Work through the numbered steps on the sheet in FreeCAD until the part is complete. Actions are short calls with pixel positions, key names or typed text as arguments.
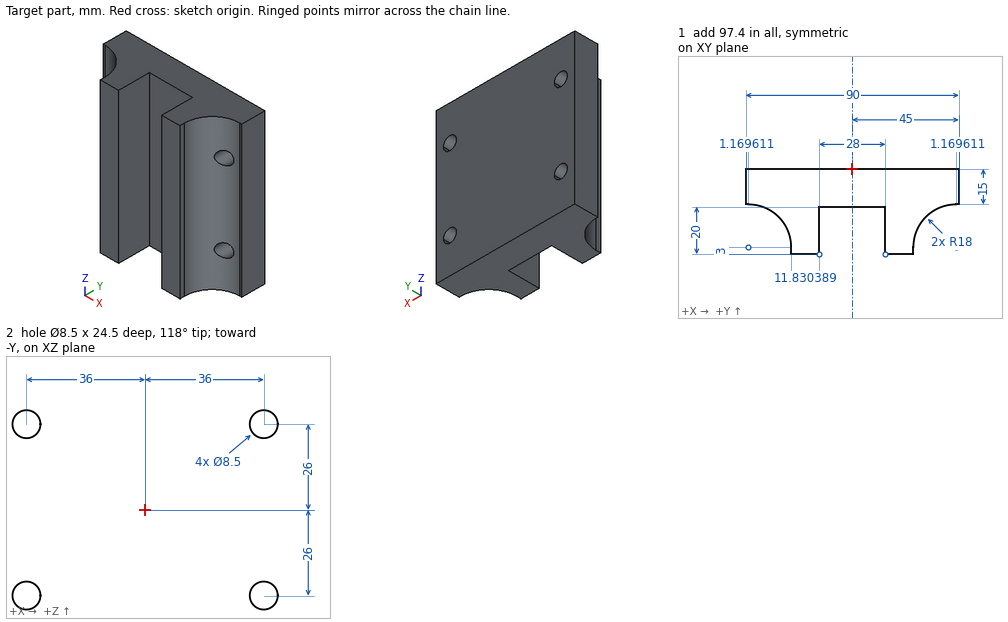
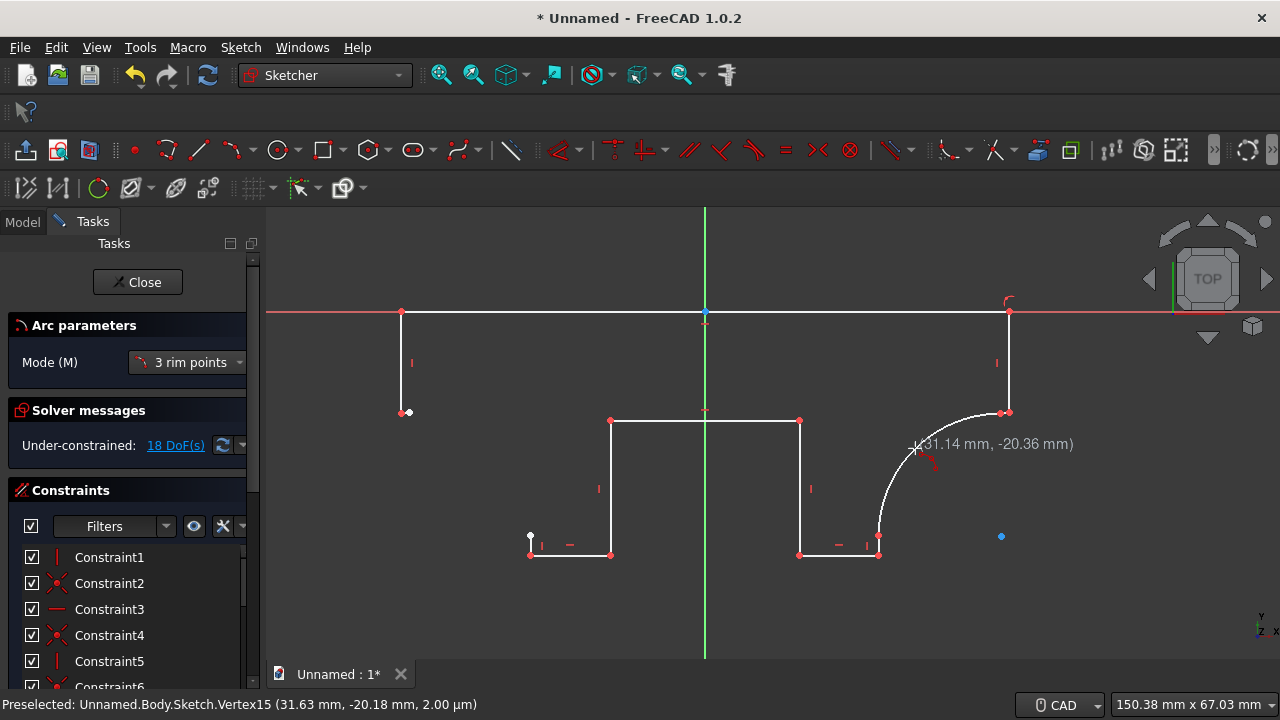
scroll(409, 413, up, 7)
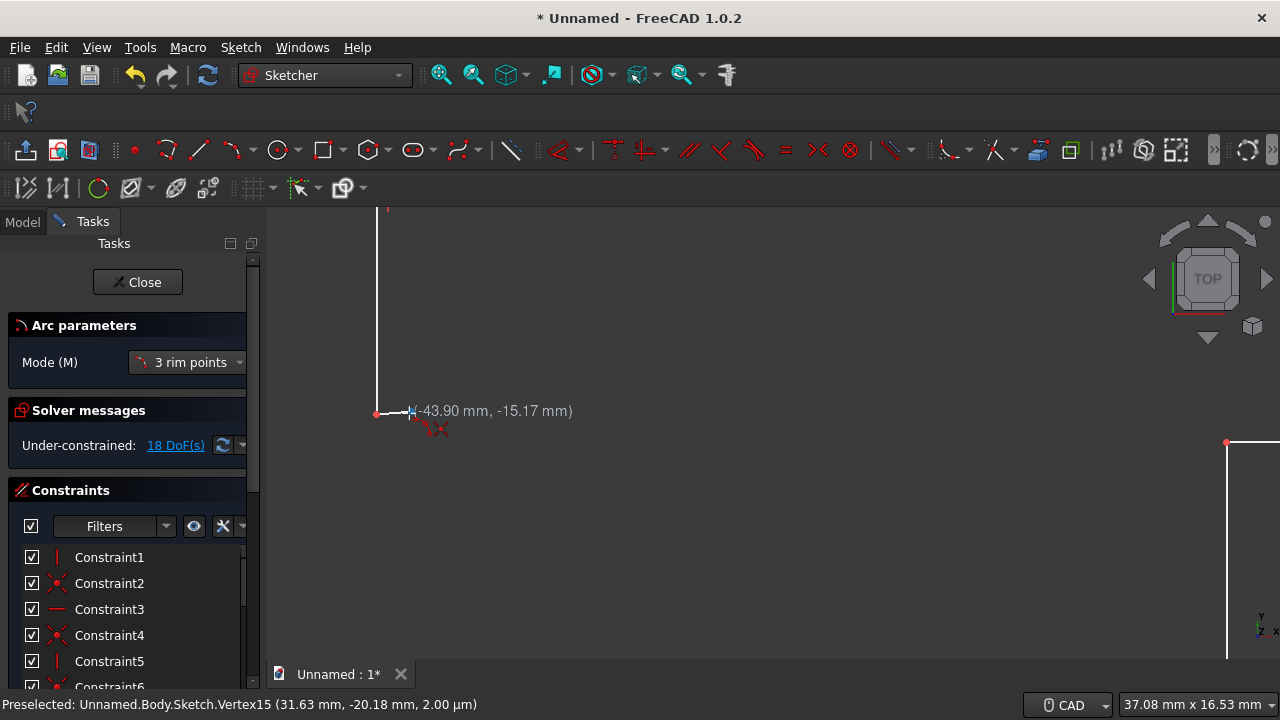
click(411, 412)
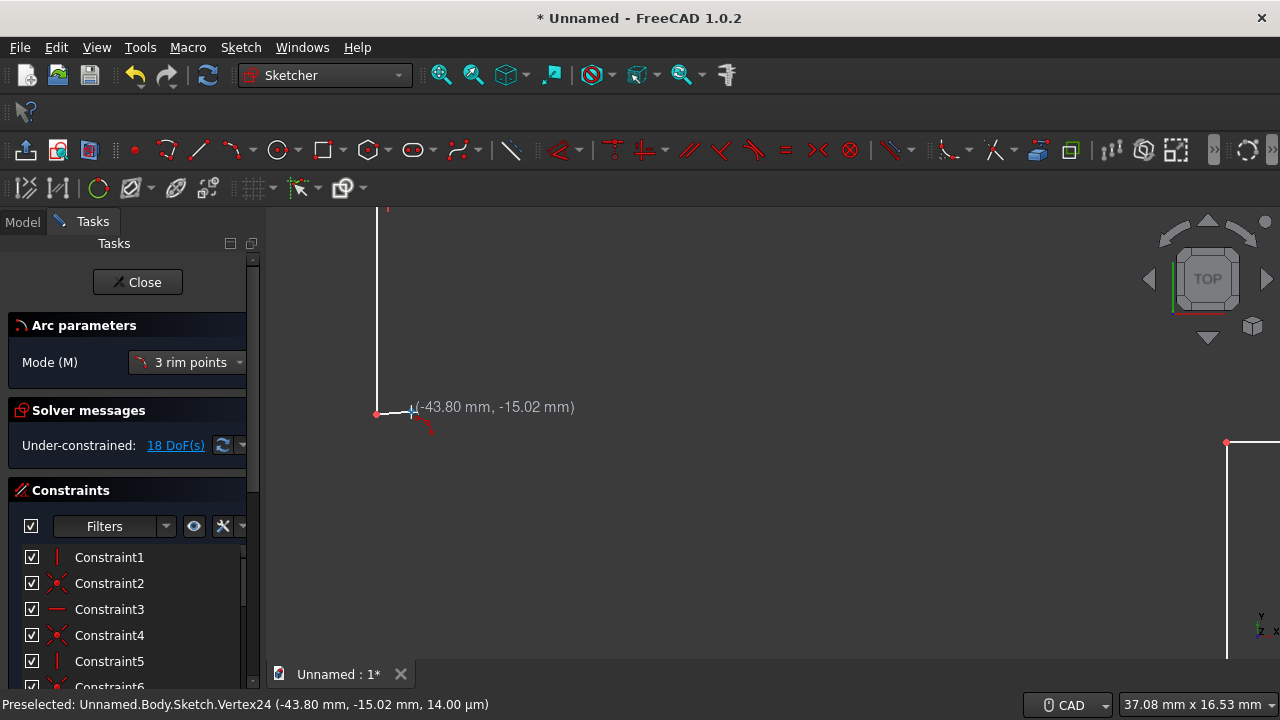
scroll(408, 413, down, 7)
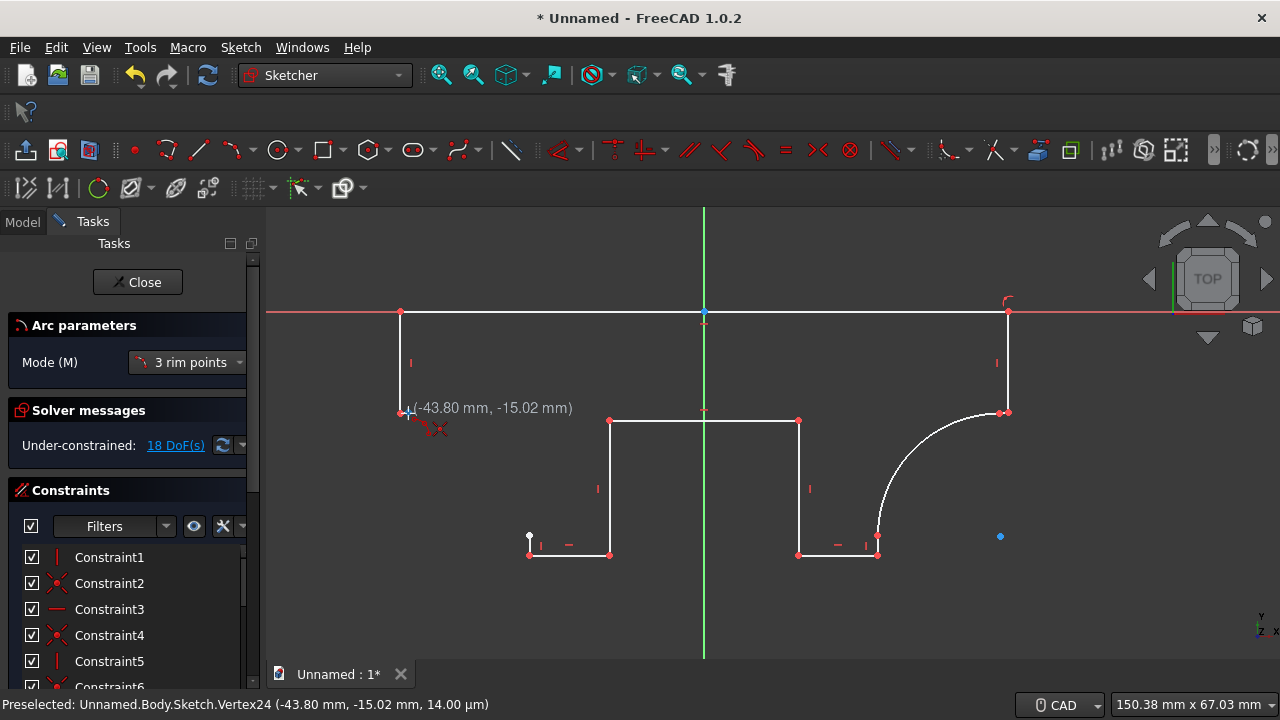
scroll(530, 534, up, 3)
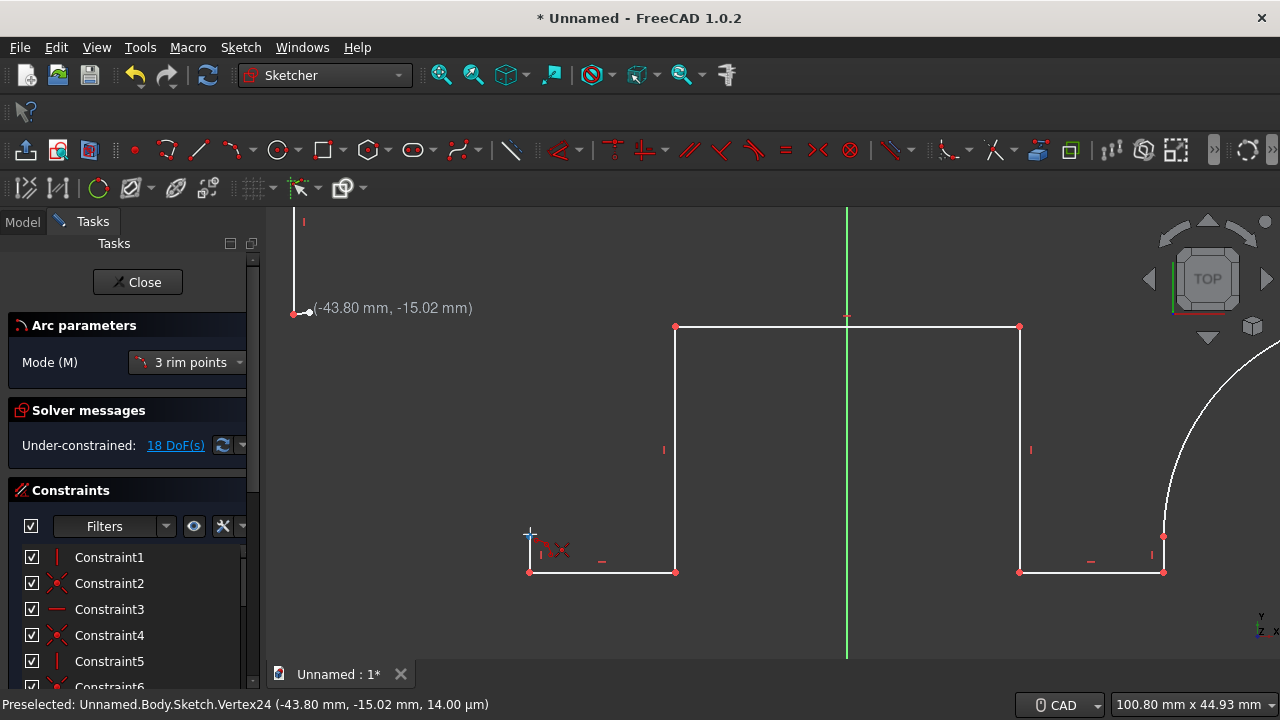
click(530, 536)
click(465, 377)
key(Escape)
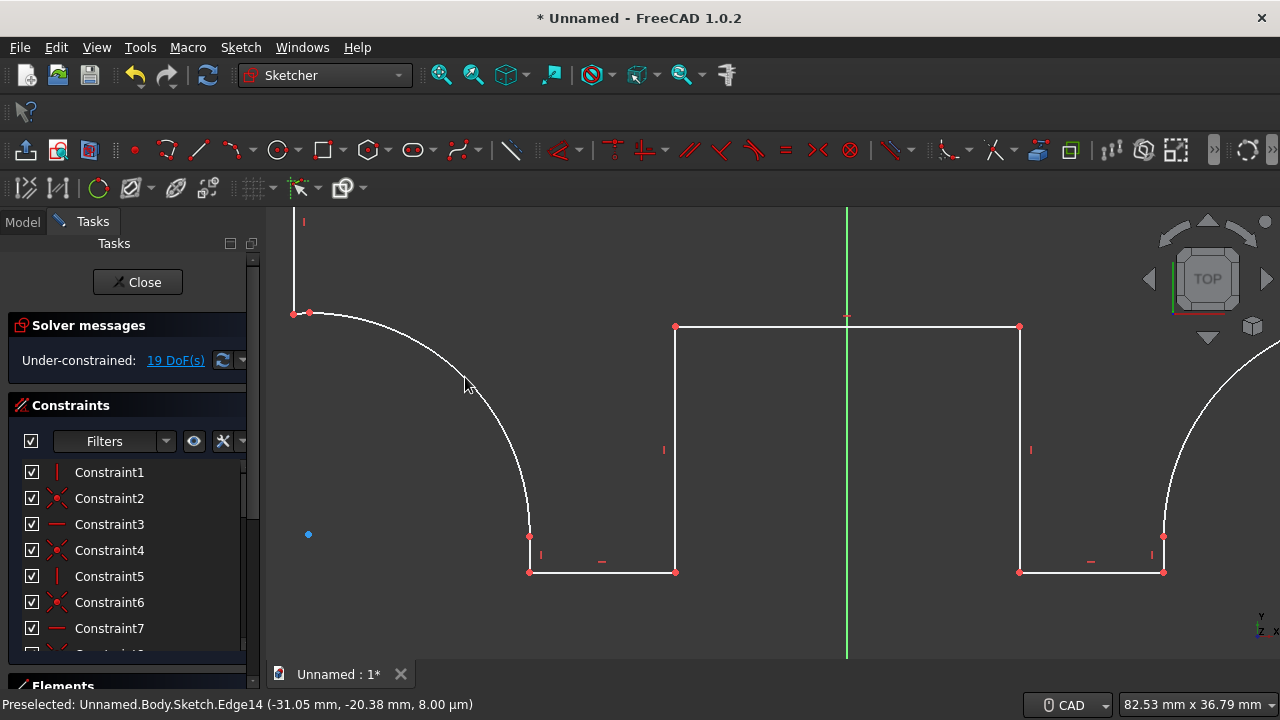
scroll(530, 547, up, 2)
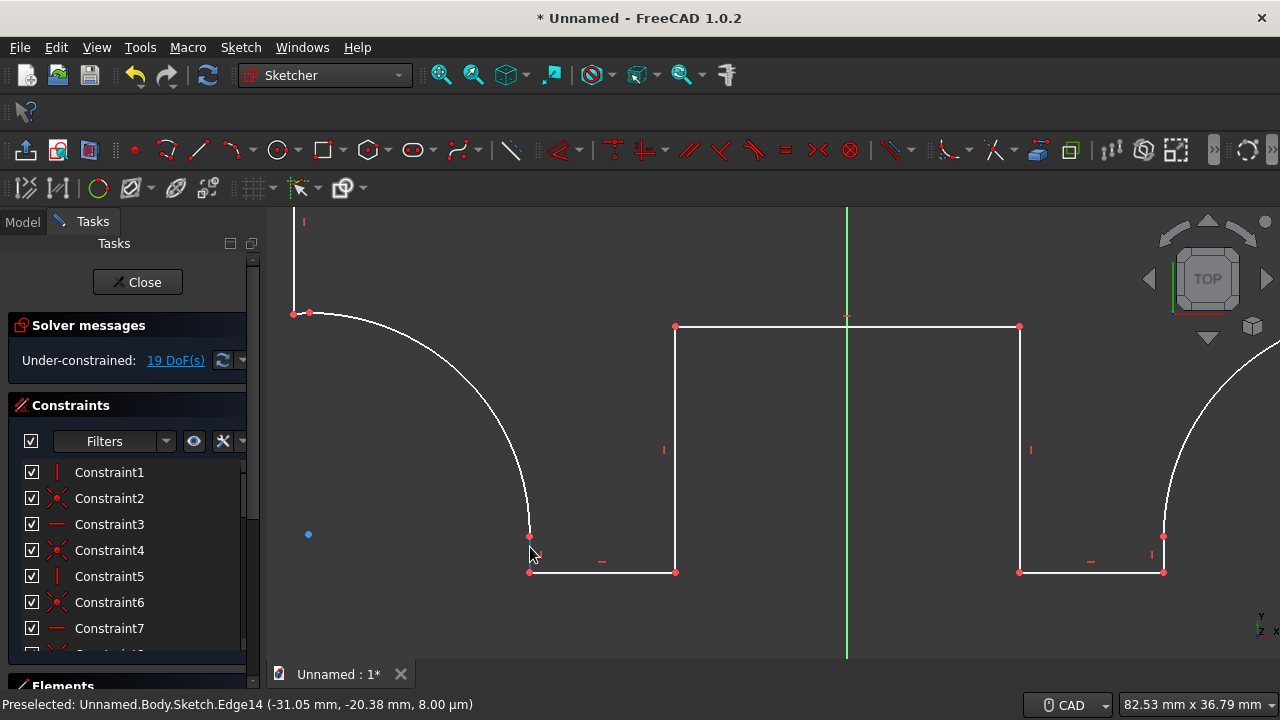
click(529, 547)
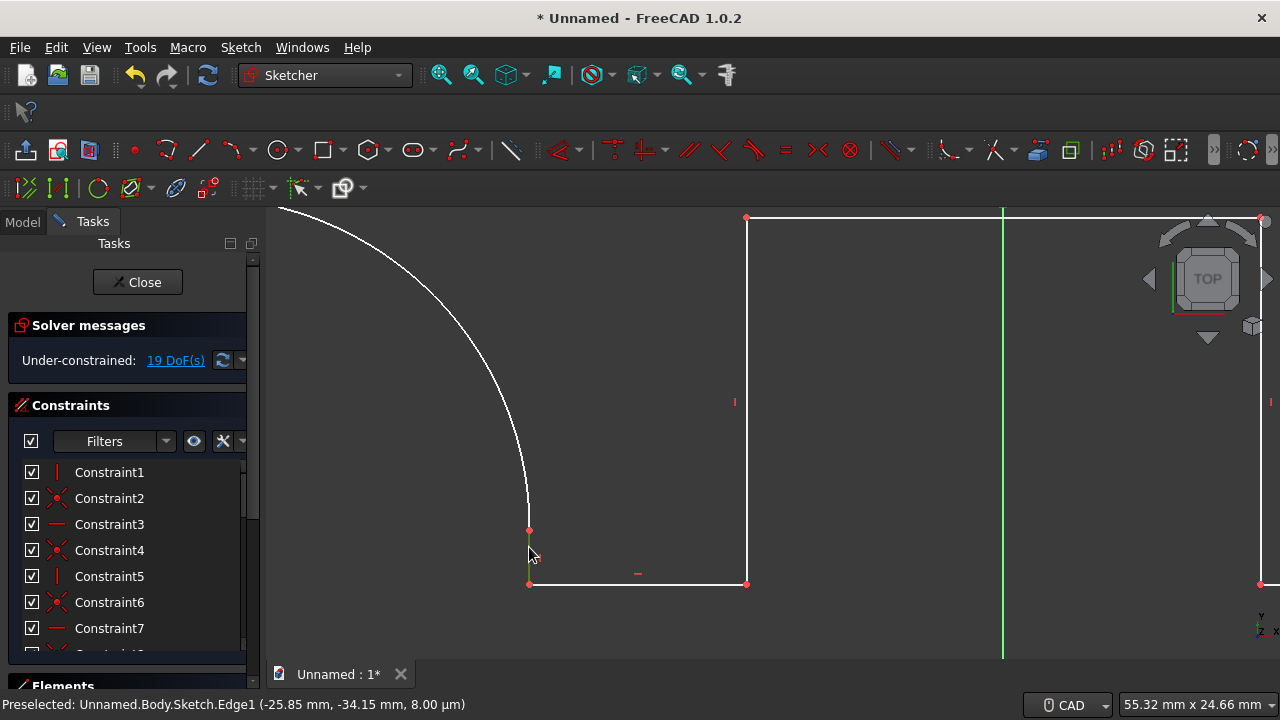
click(494, 380)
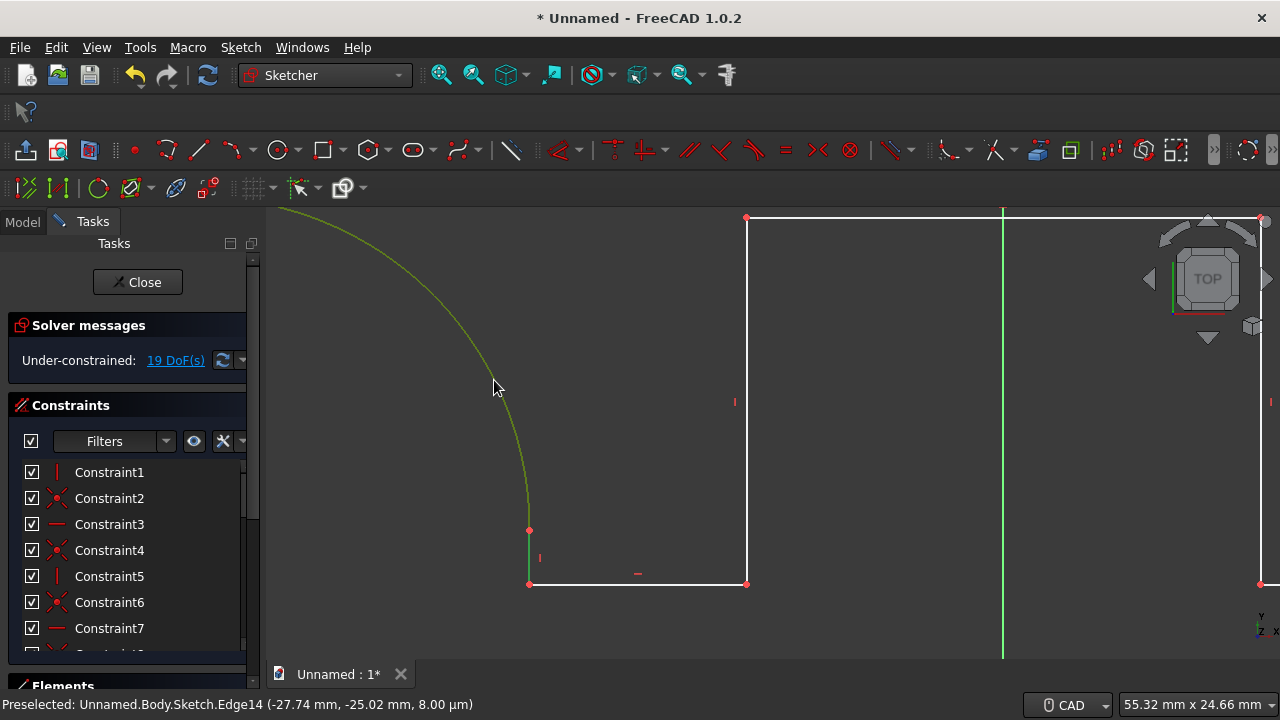
click(754, 150)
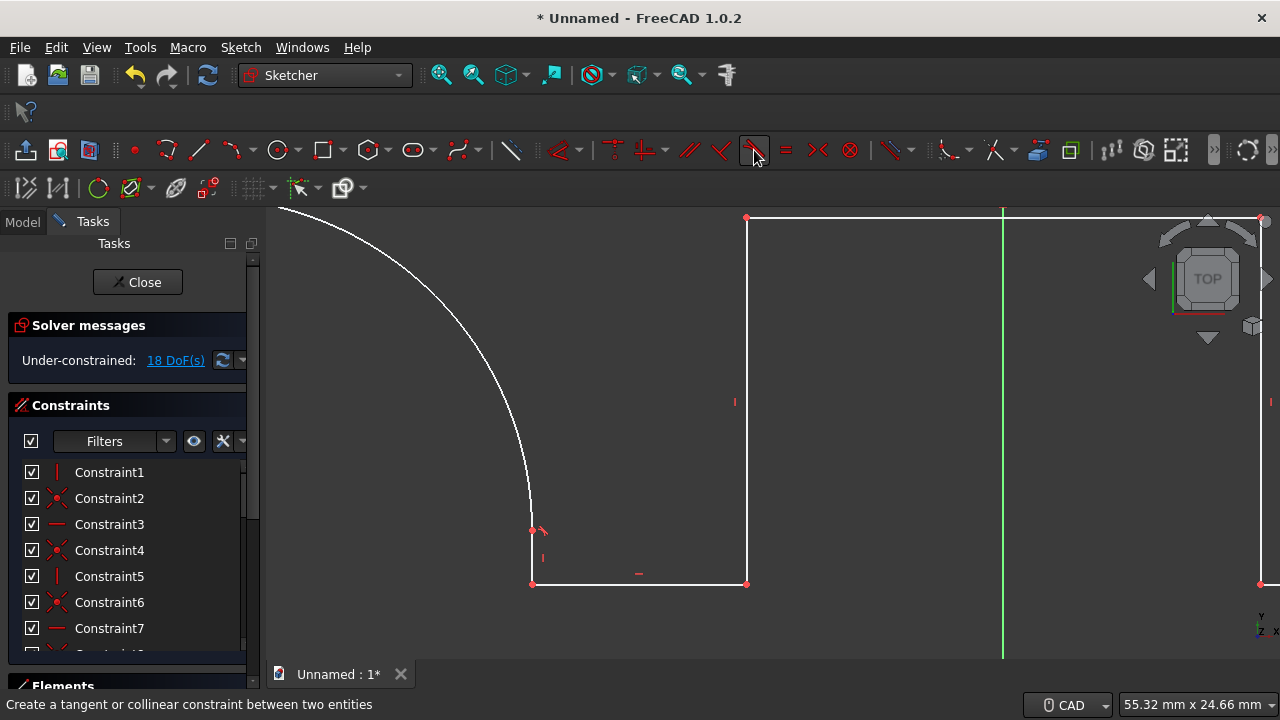
scroll(531, 538, down, 5)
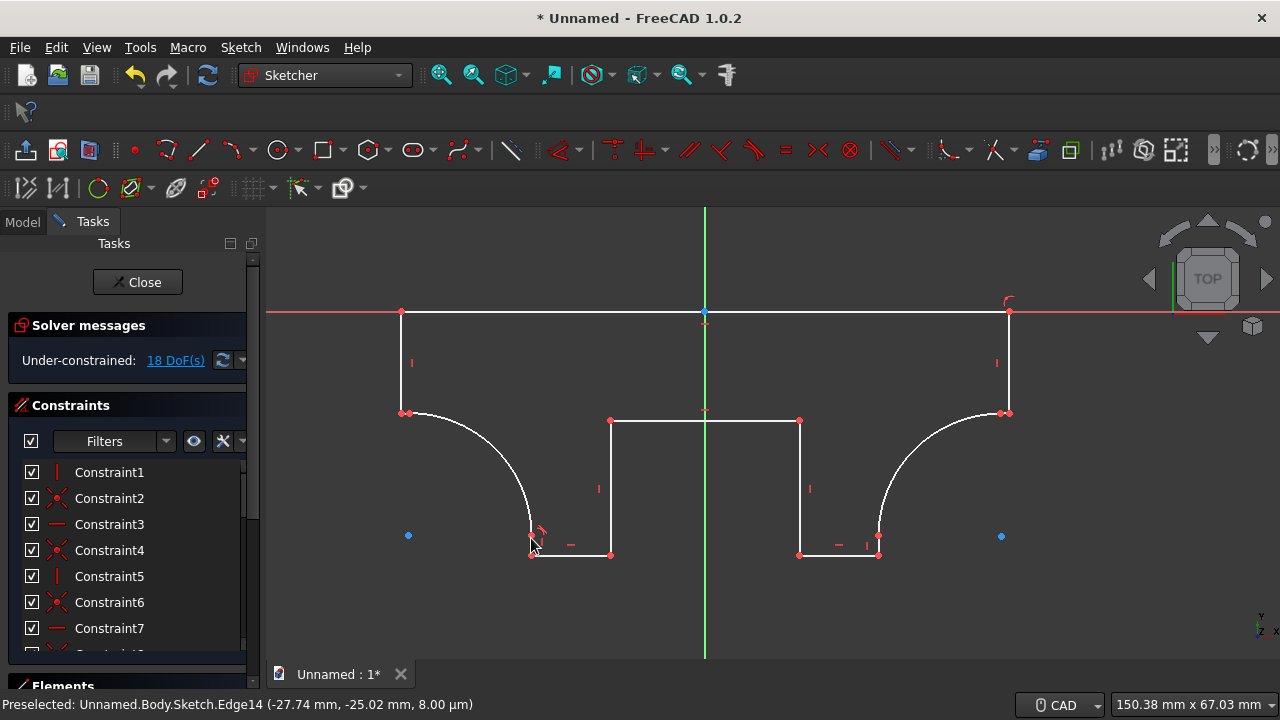
scroll(879, 550, up, 5)